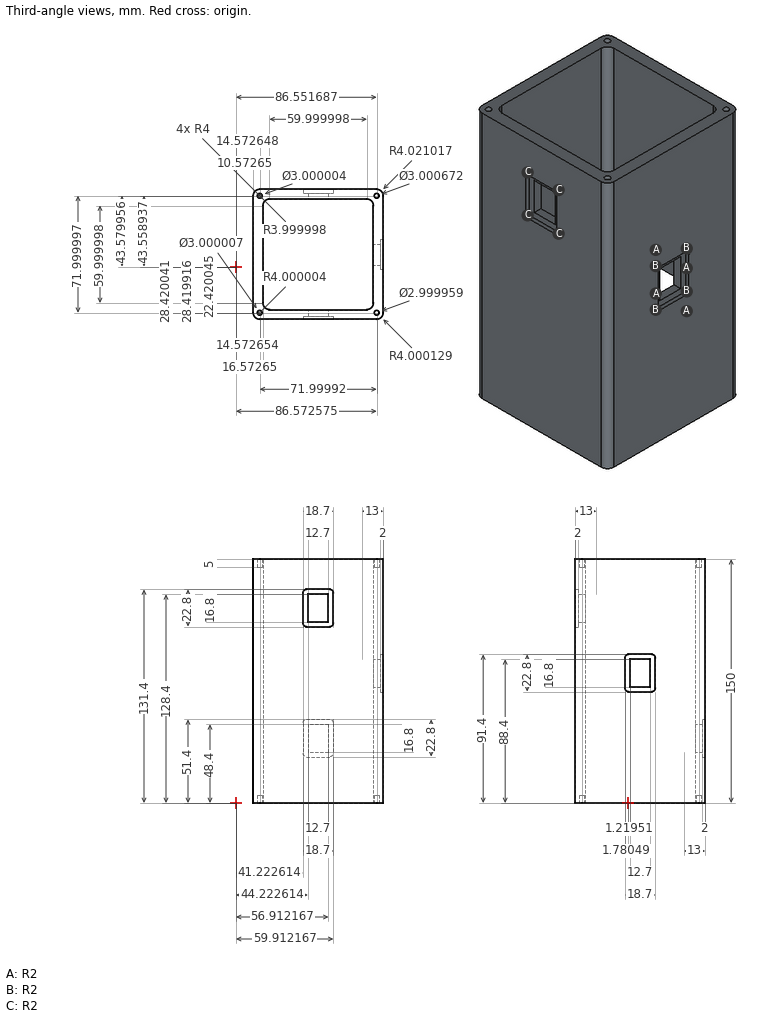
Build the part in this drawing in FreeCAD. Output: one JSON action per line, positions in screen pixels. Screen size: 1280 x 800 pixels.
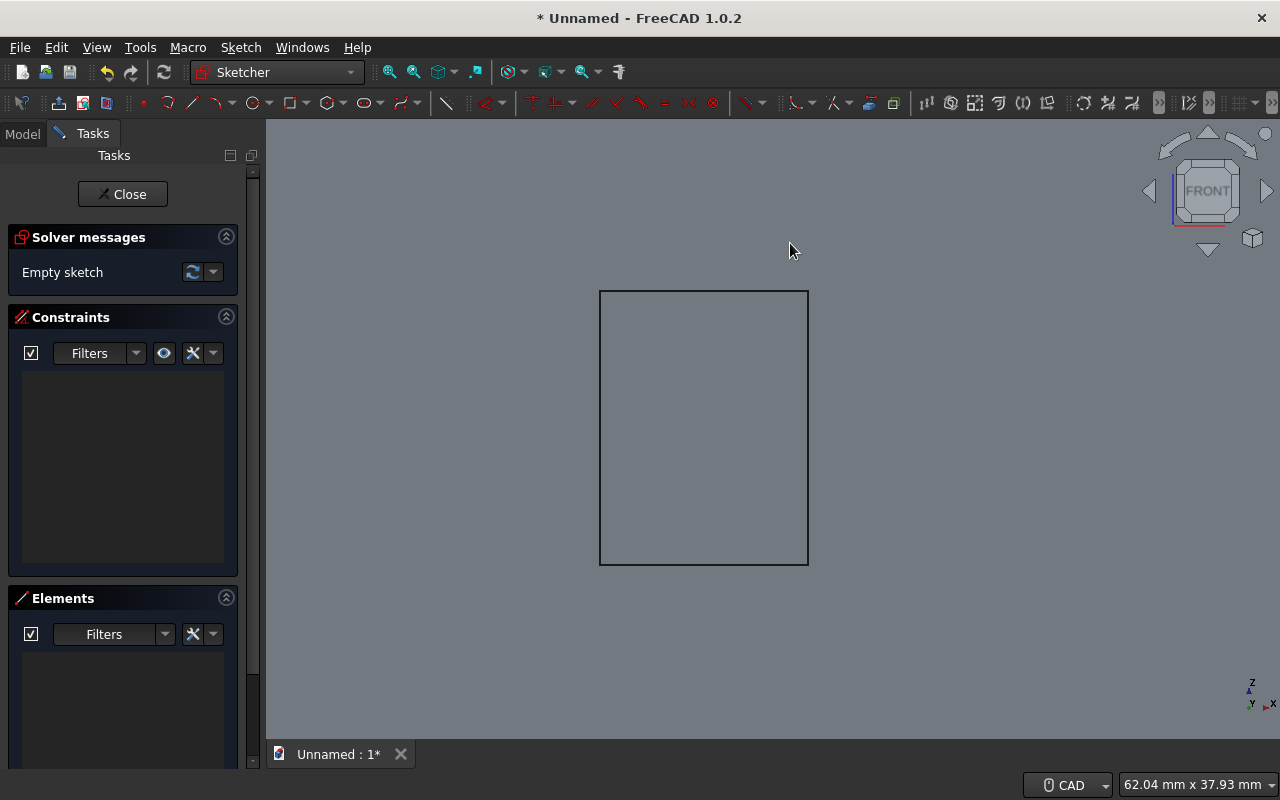
{"action": "left_click", "coordinate": [290, 104]}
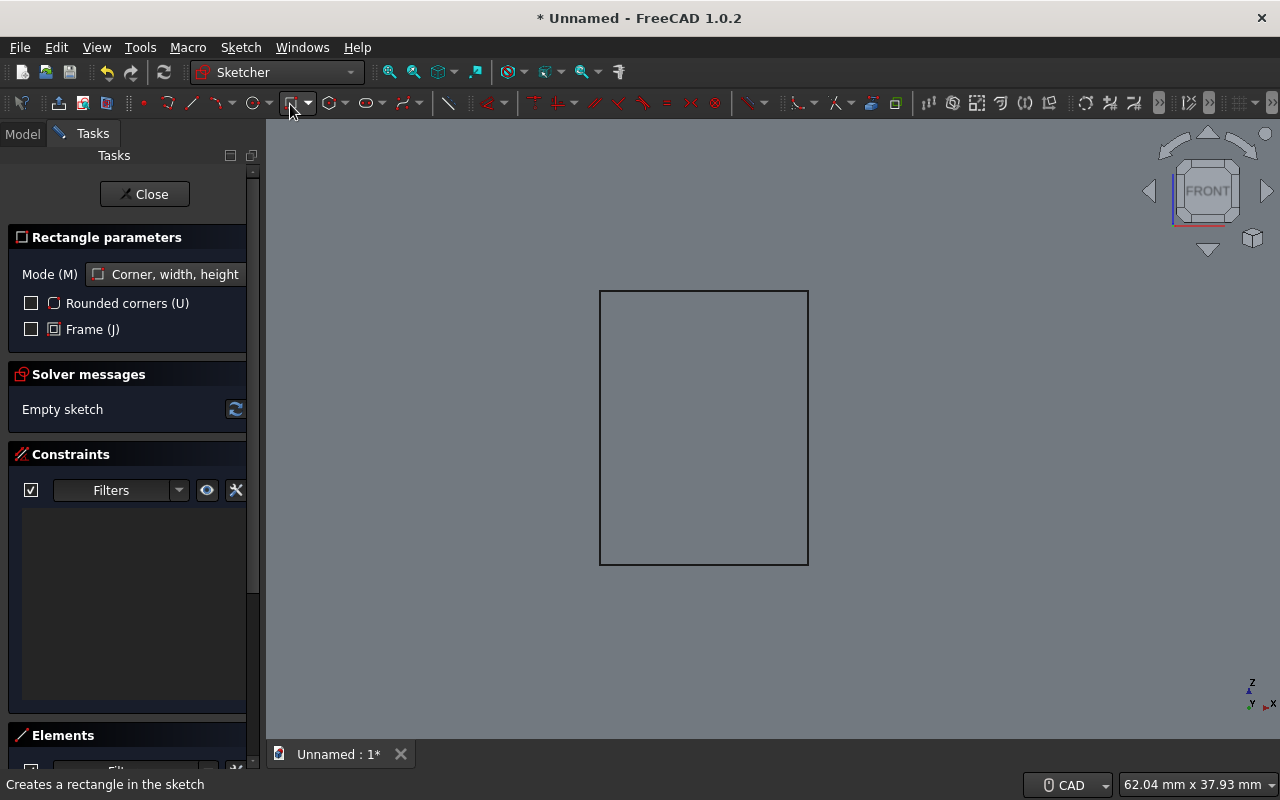
{"action": "left_click", "coordinate": [551, 242]}
{"action": "left_click", "coordinate": [857, 614]}
{"action": "key", "text": "Escape"}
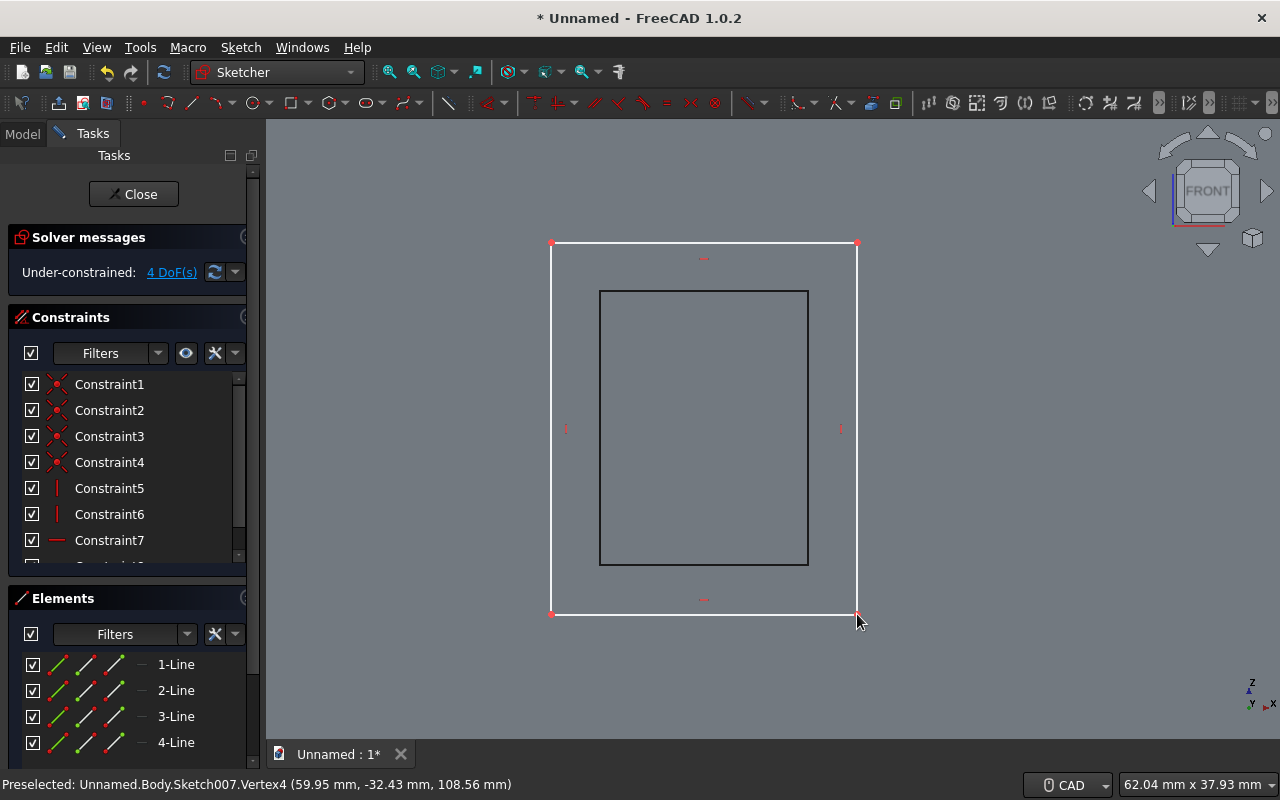
{"action": "left_click", "coordinate": [488, 104]}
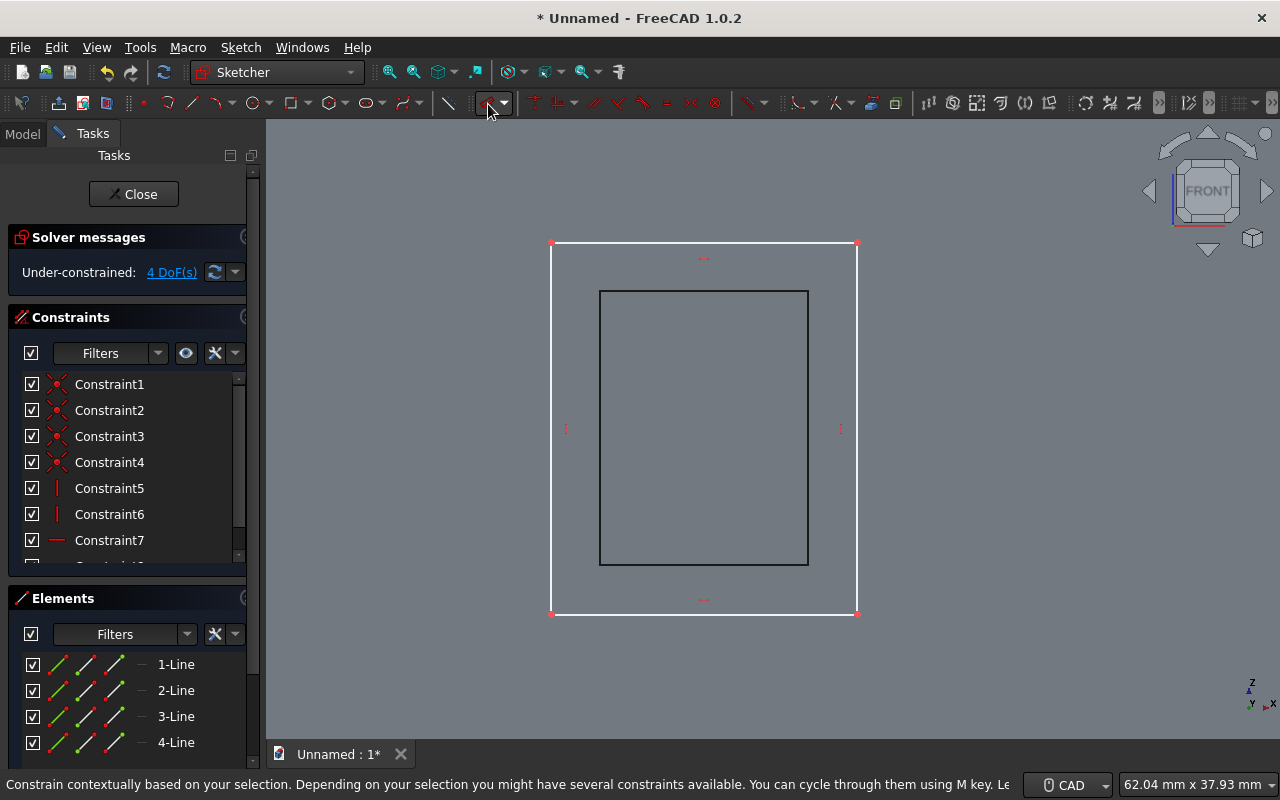
{"action": "left_click", "coordinate": [551, 355]}
{"action": "left_click", "coordinate": [517, 429]}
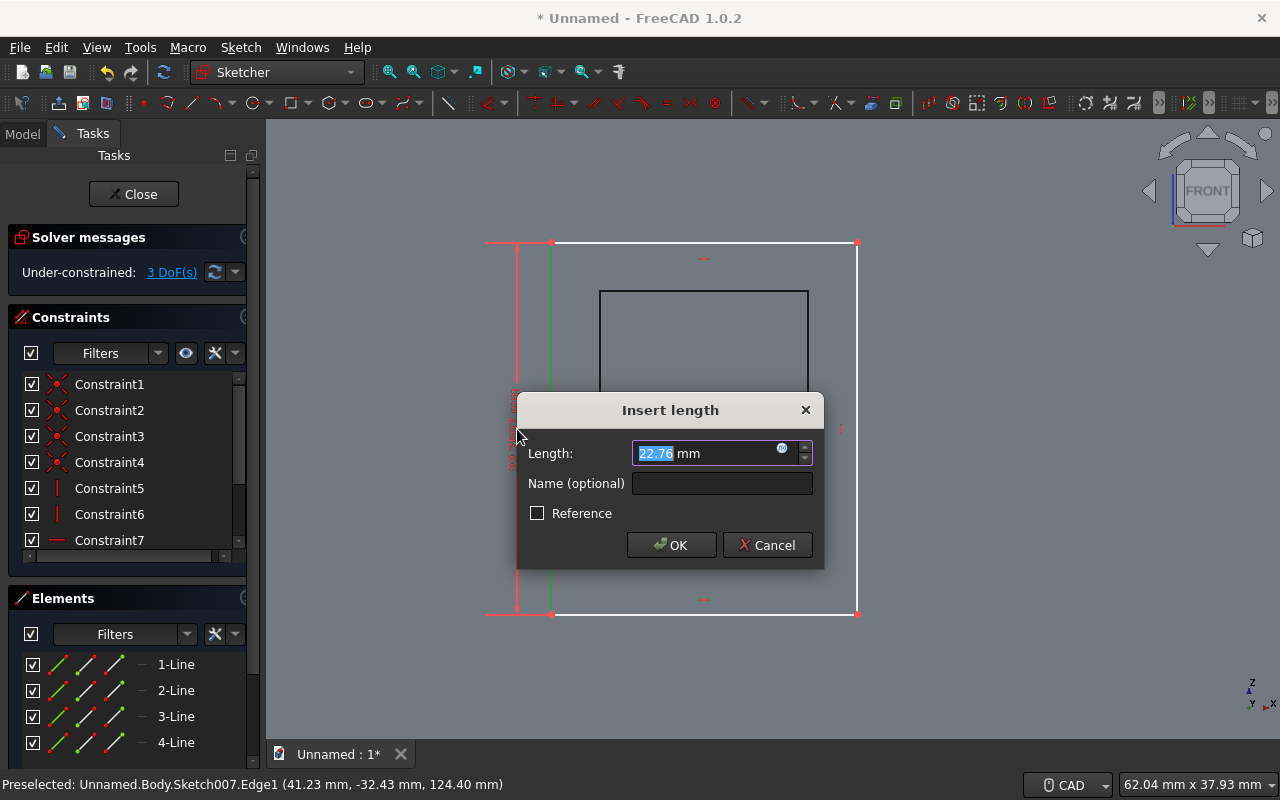
{"action": "type", "text": "22.8"}
{"action": "key", "text": "Return"}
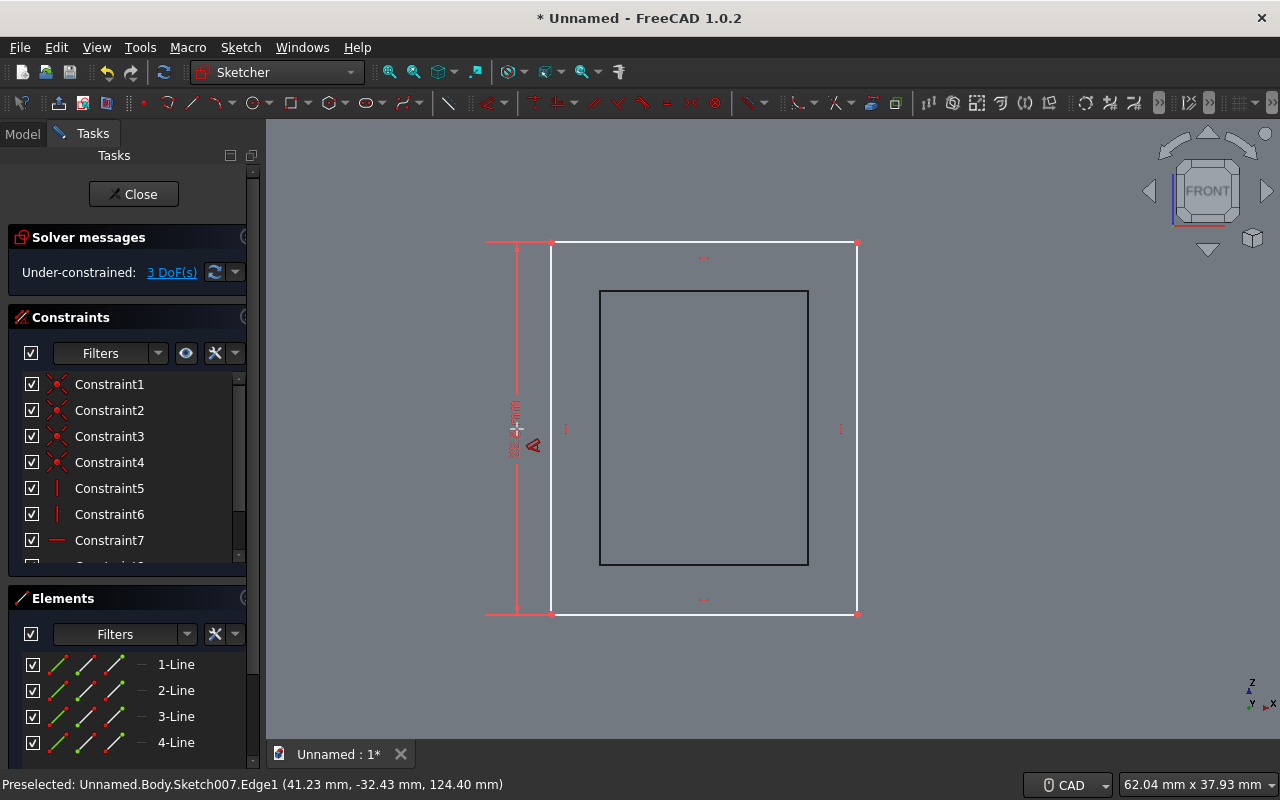
{"action": "left_click", "coordinate": [643, 615]}
{"action": "left_click", "coordinate": [704, 649]}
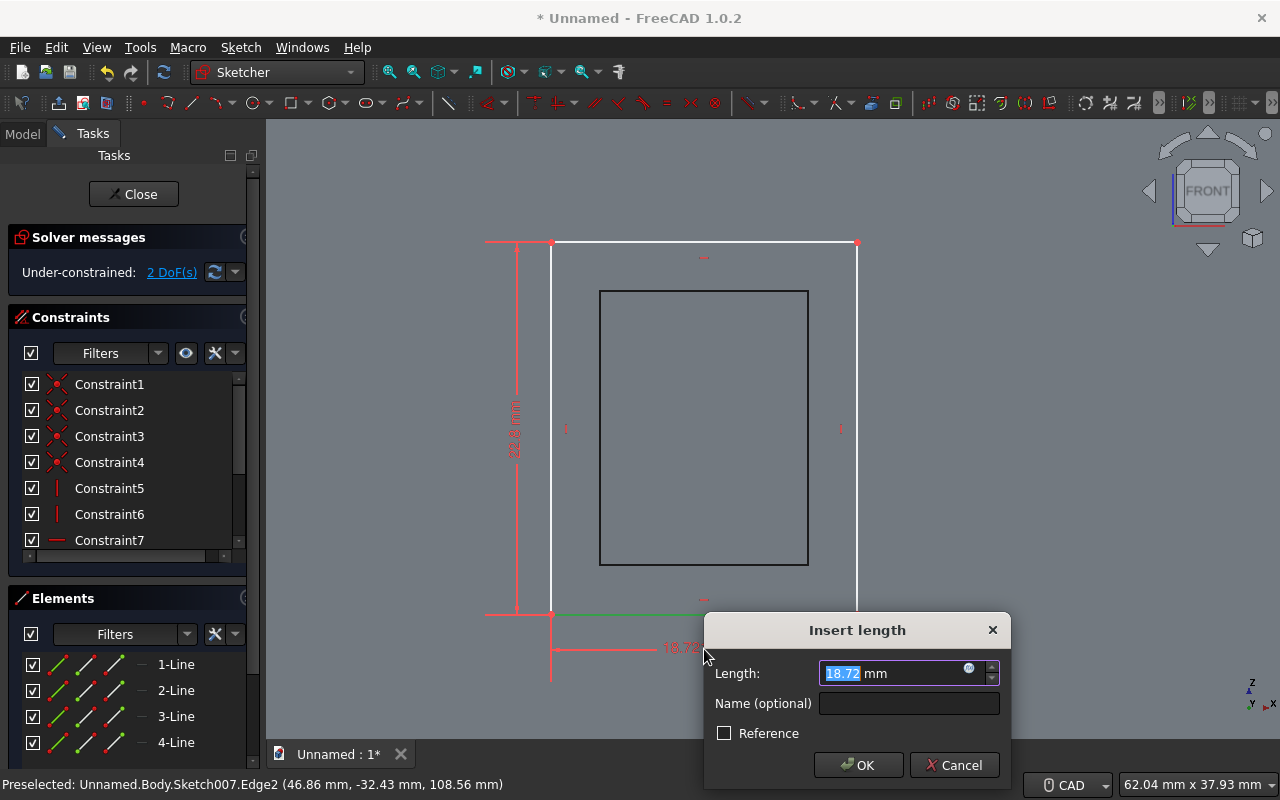
{"action": "type", "text": "18.7"}
{"action": "key", "text": "Return"}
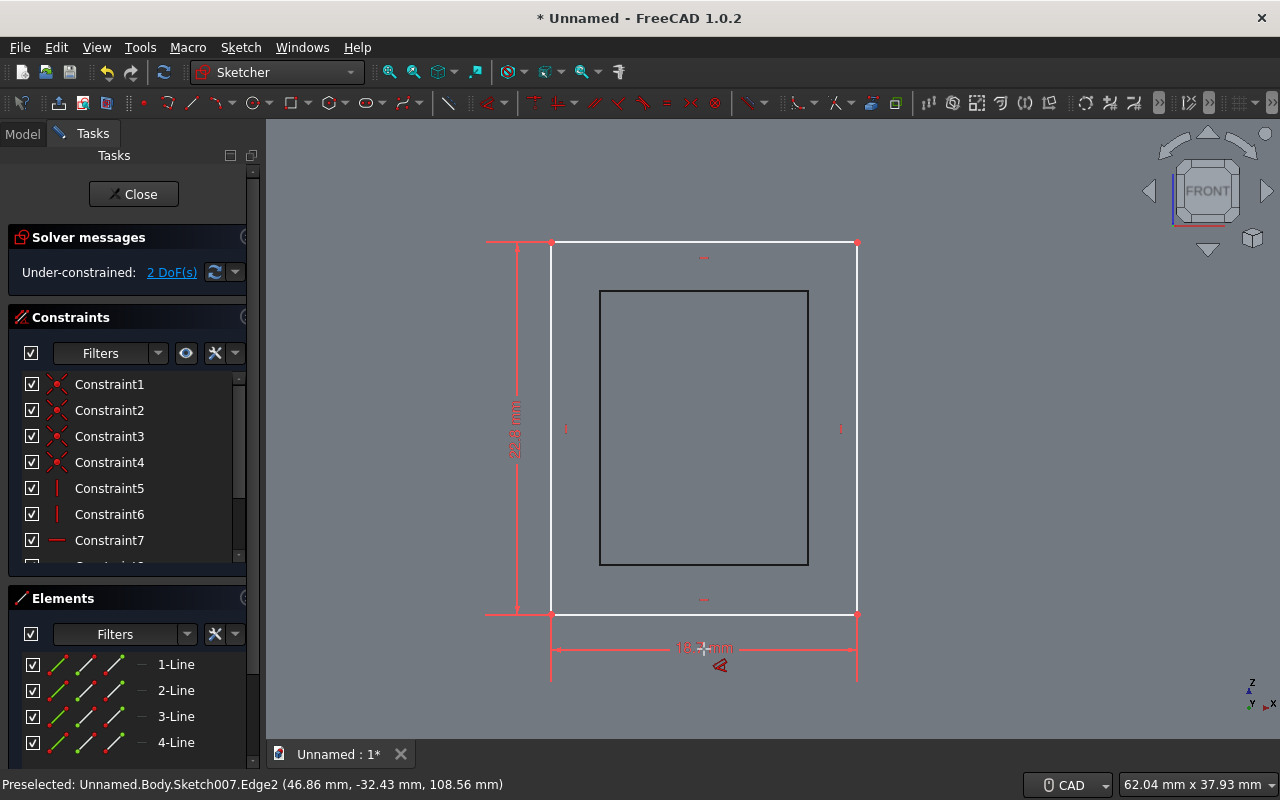
{"action": "left_click", "coordinate": [551, 242]}
{"action": "left_click", "coordinate": [585, 477]}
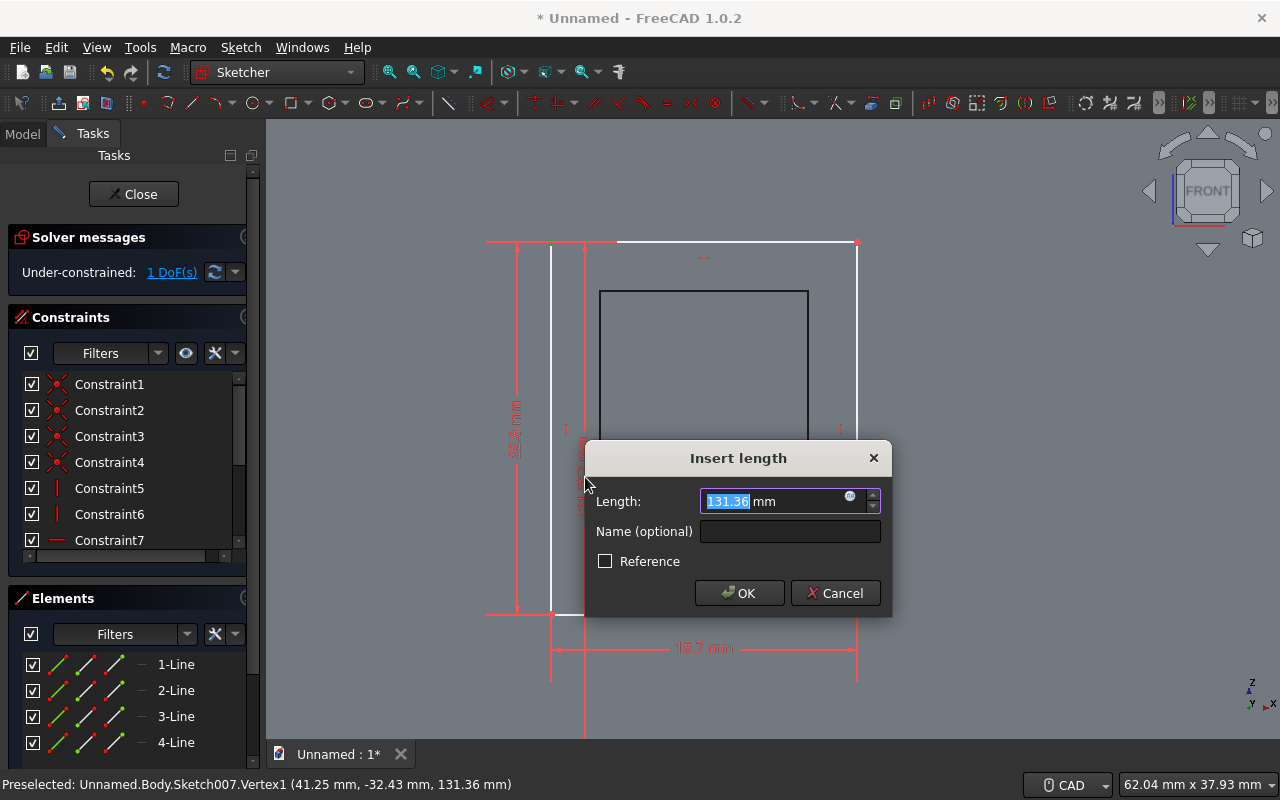
{"action": "type", "text": "131.4"}
{"action": "key", "text": "Return"}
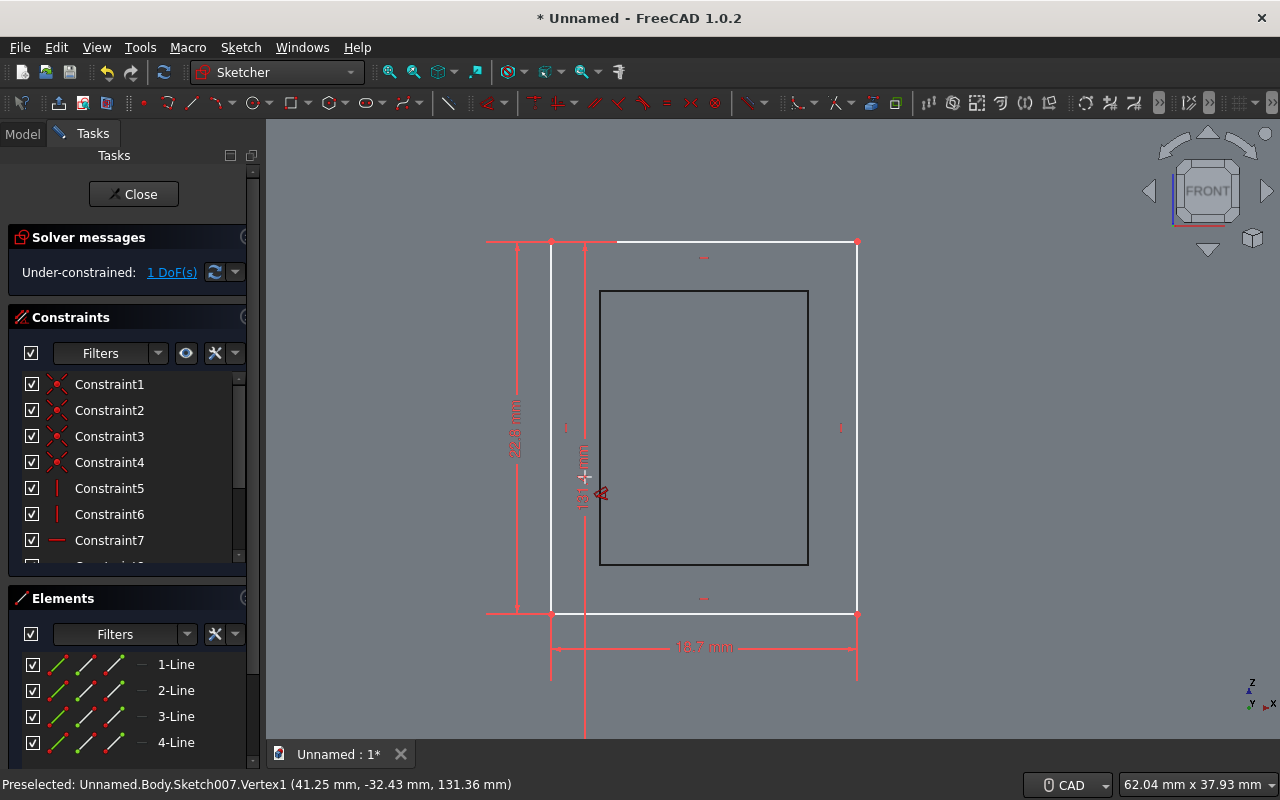
{"action": "left_click", "coordinate": [551, 242]}
{"action": "left_click", "coordinate": [423, 208]}